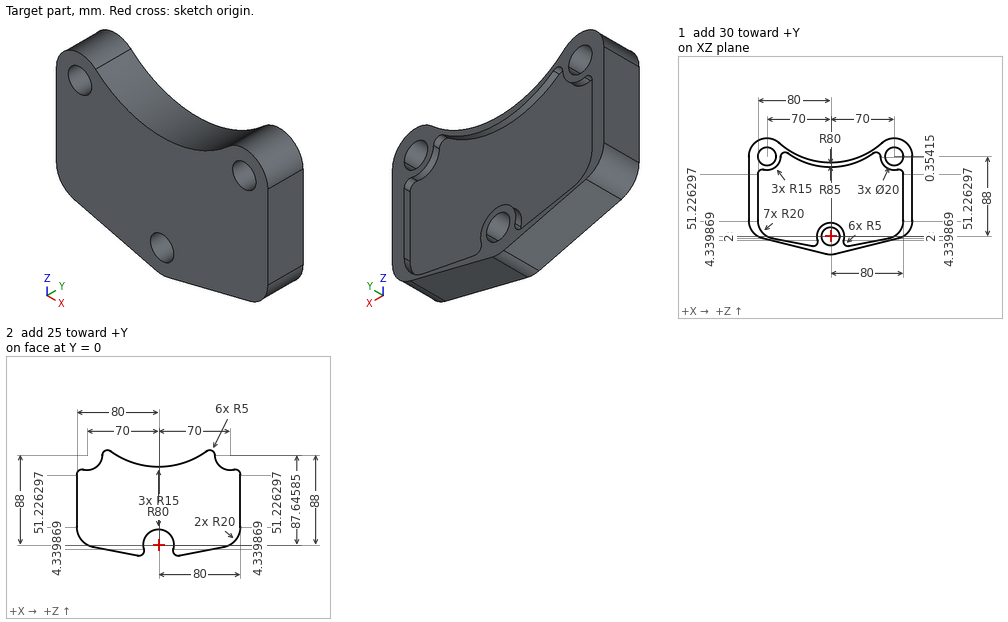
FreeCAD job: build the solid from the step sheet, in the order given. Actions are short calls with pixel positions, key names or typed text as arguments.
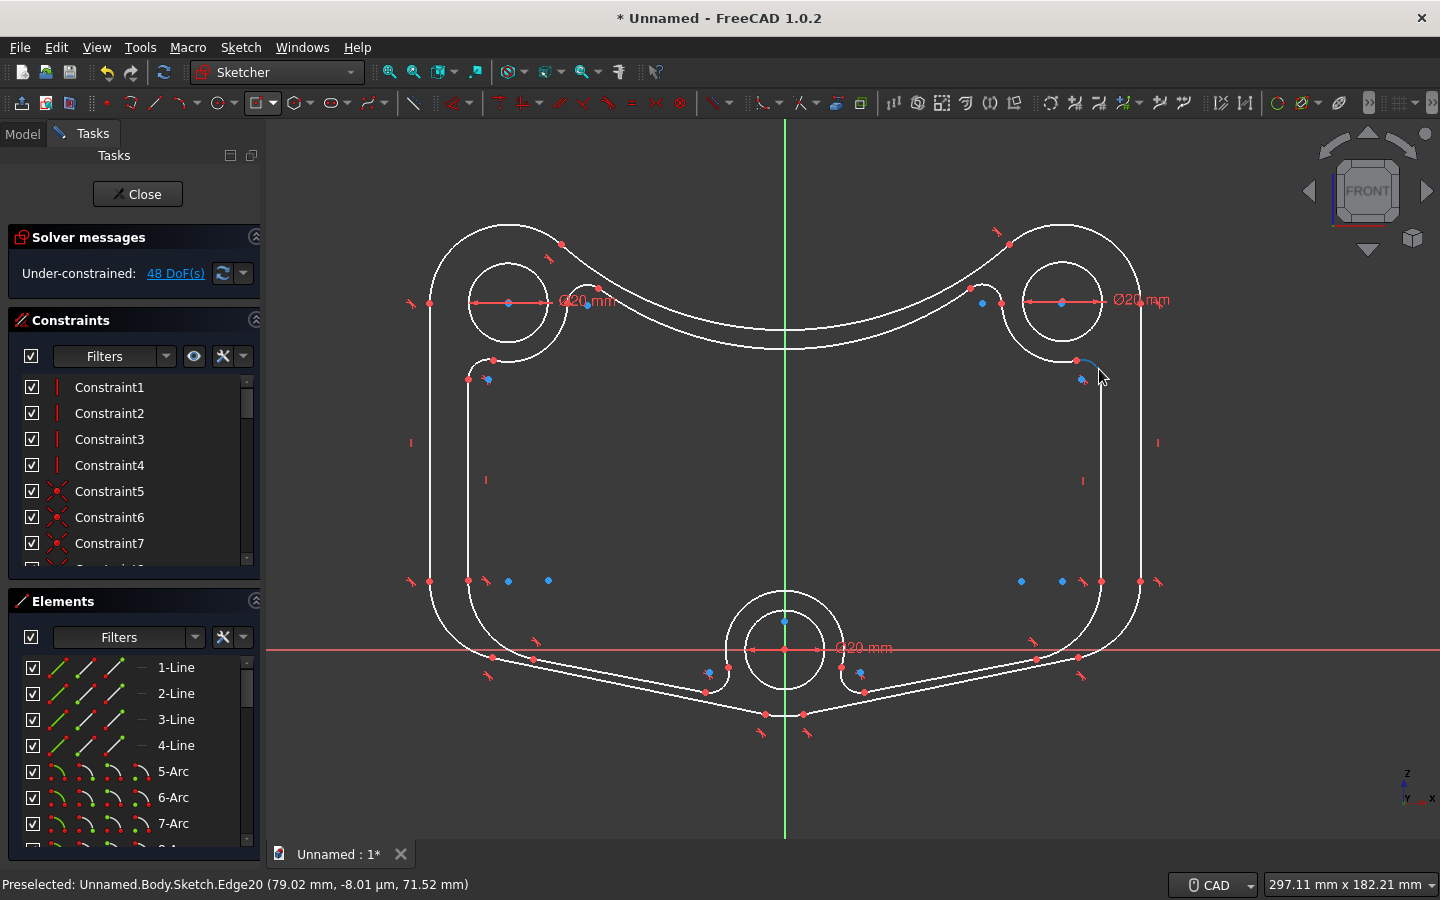
click(717, 691)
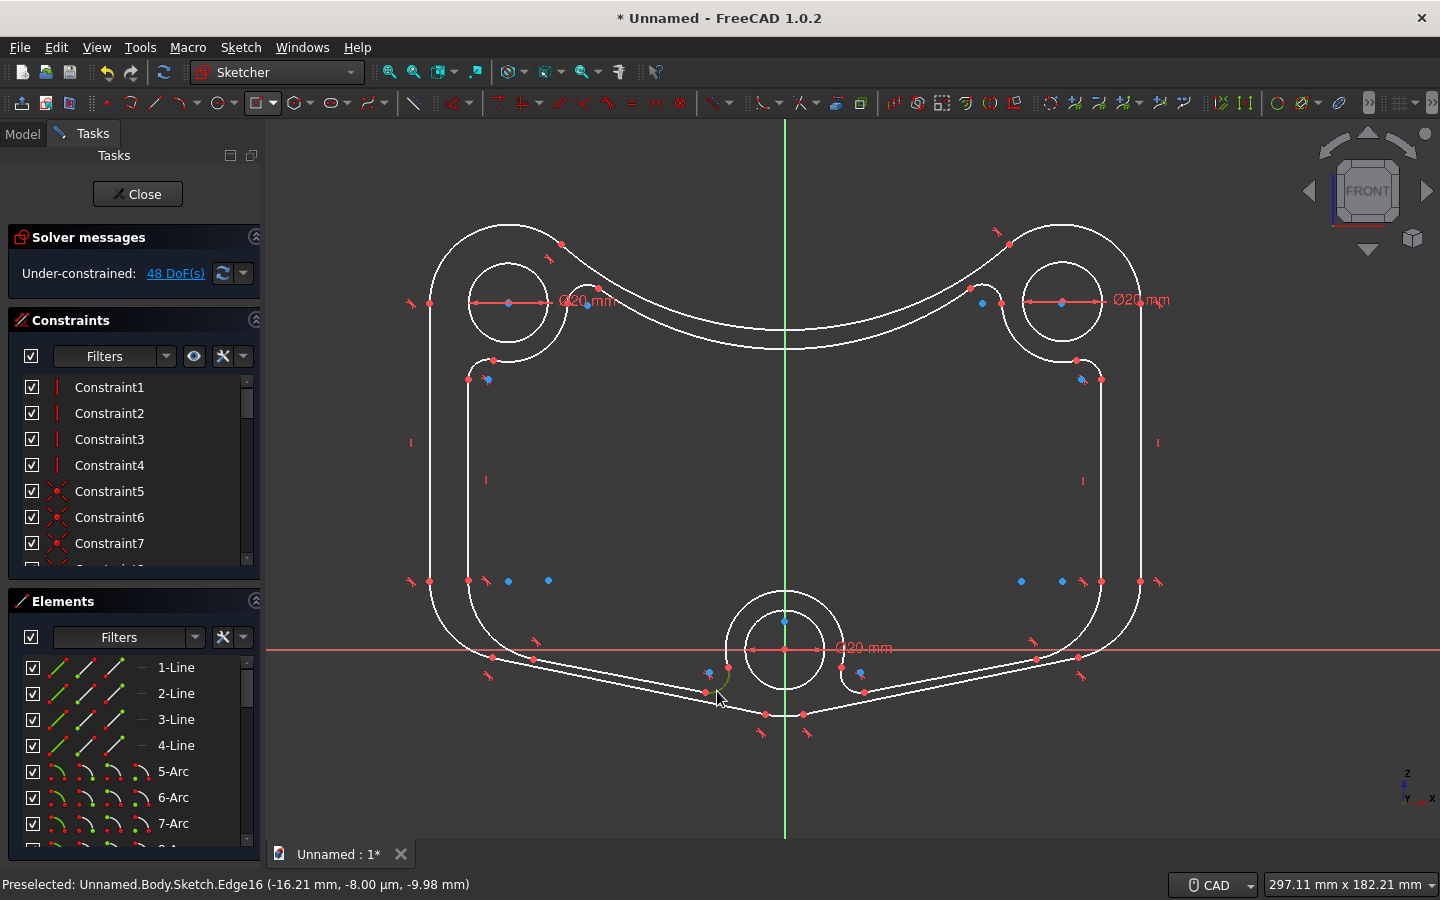
click(825, 607)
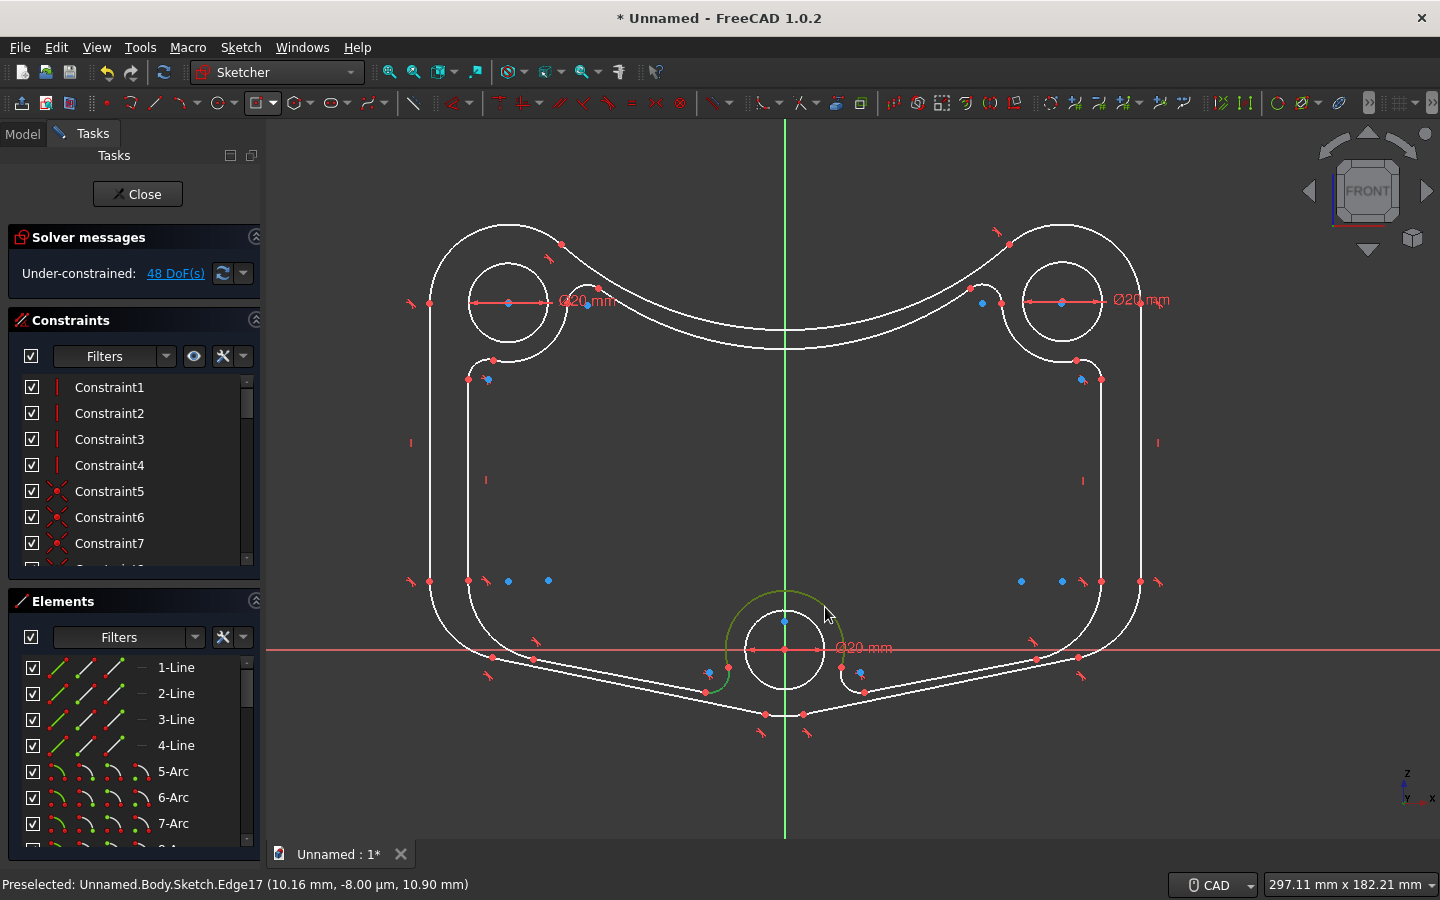
key(t)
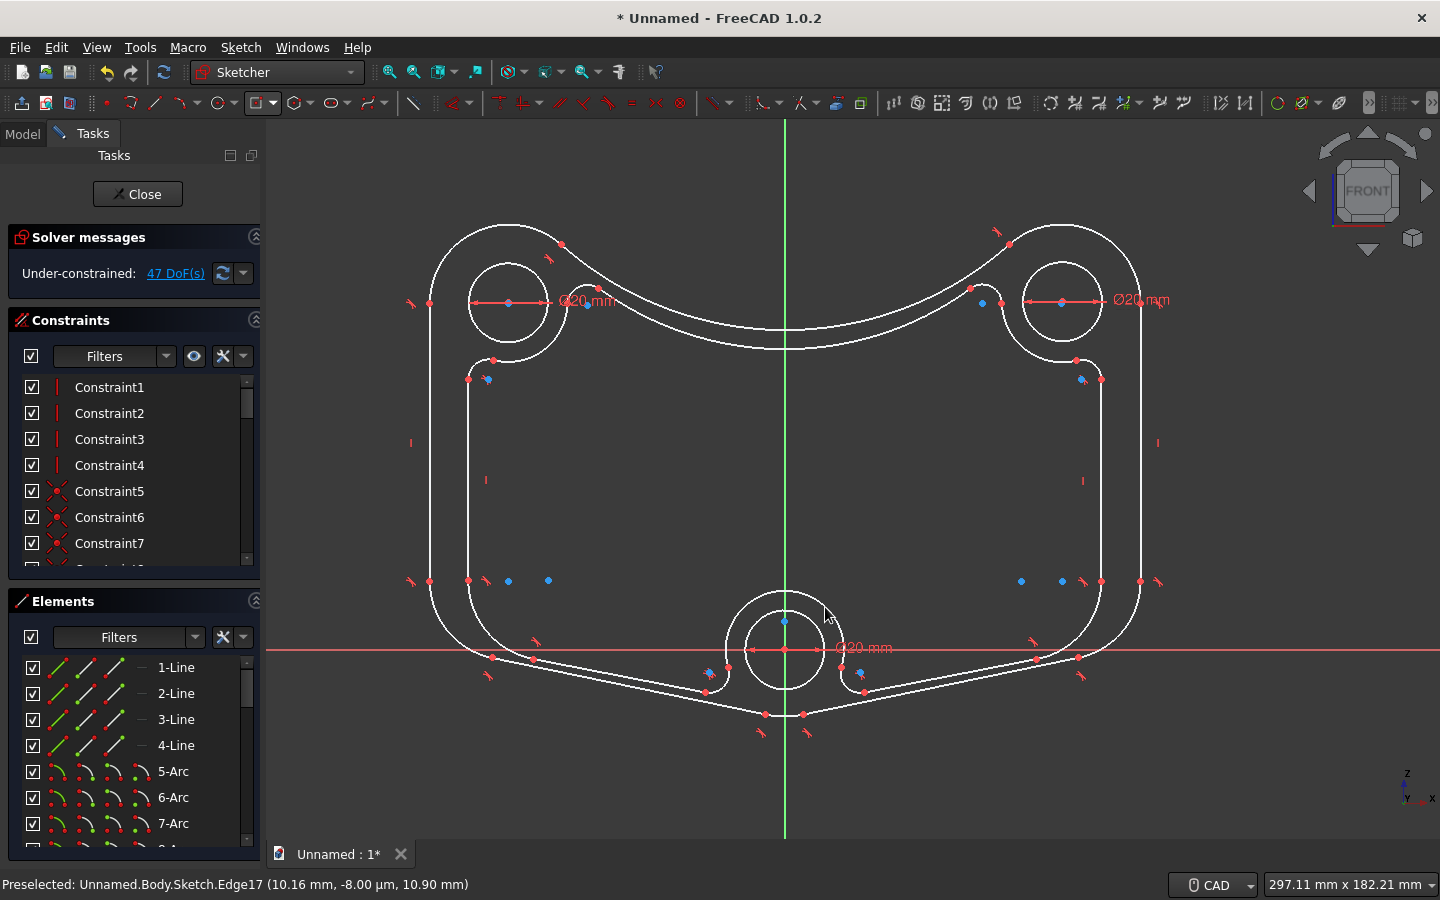
click(825, 607)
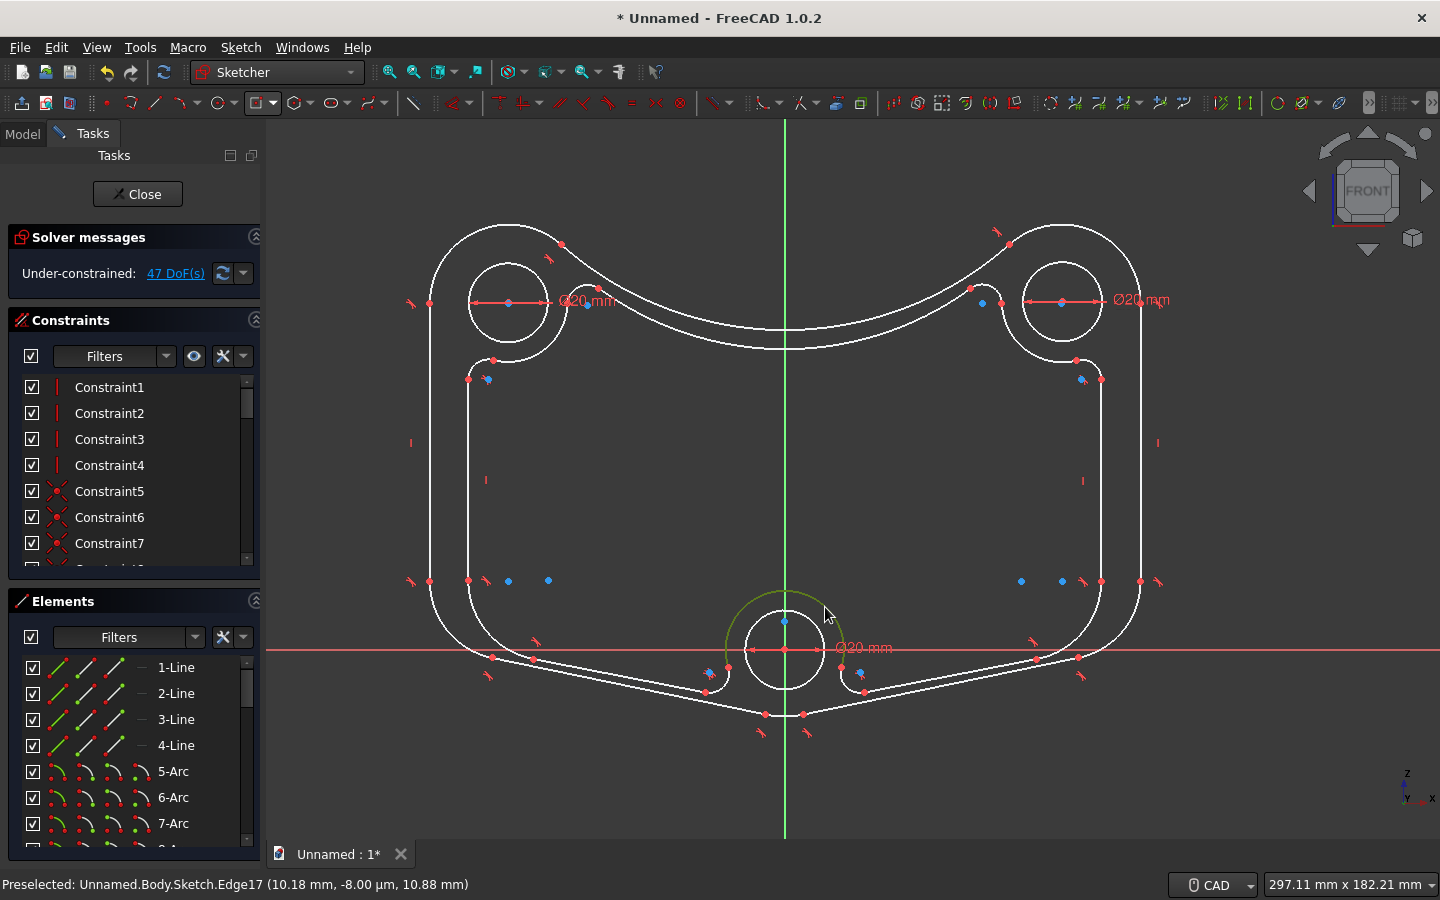
click(842, 679)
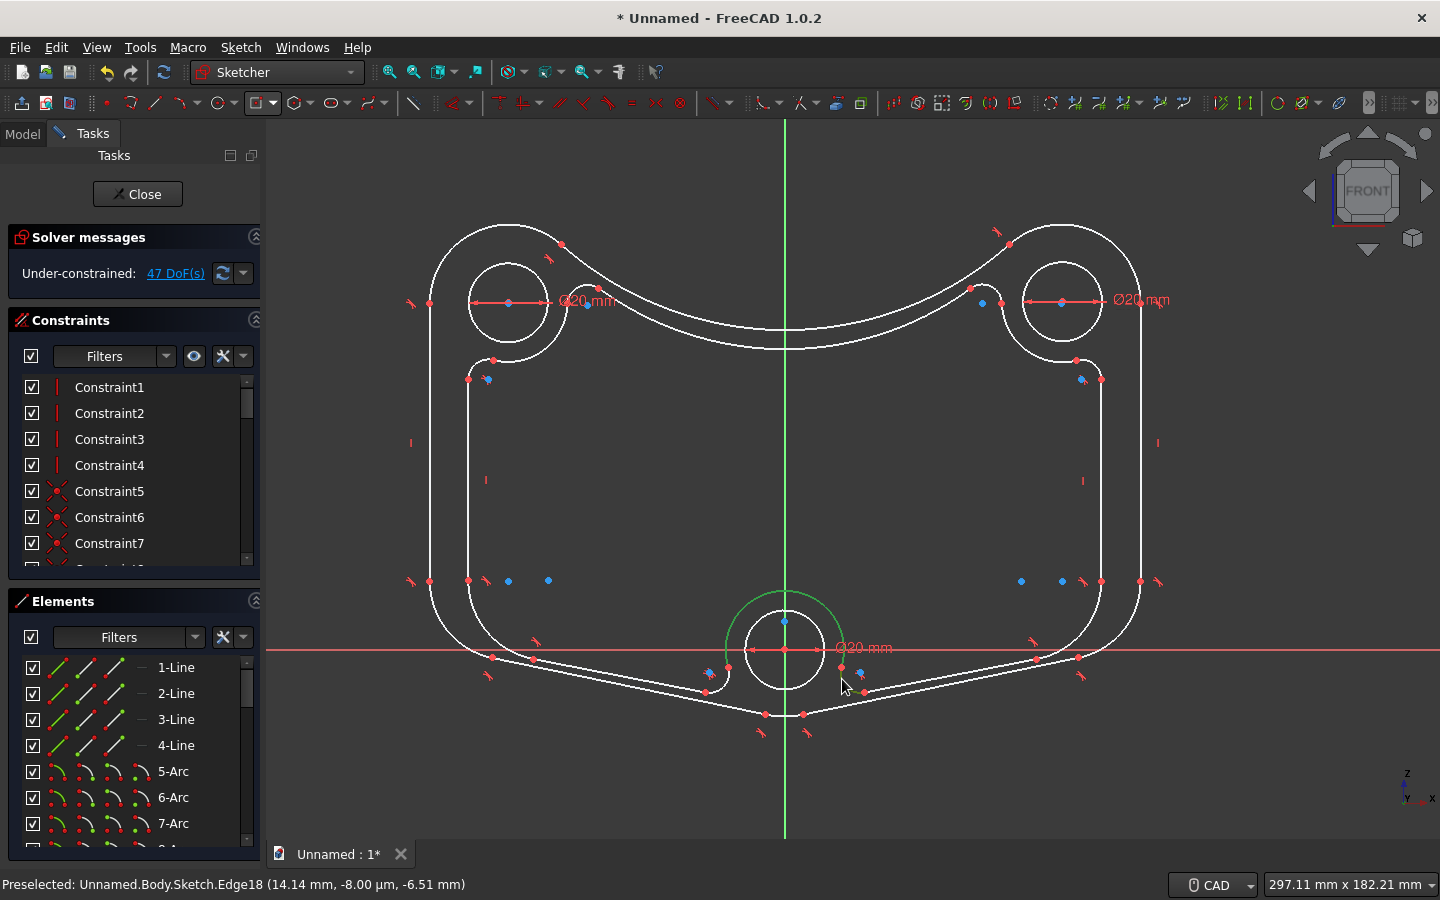
click(608, 104)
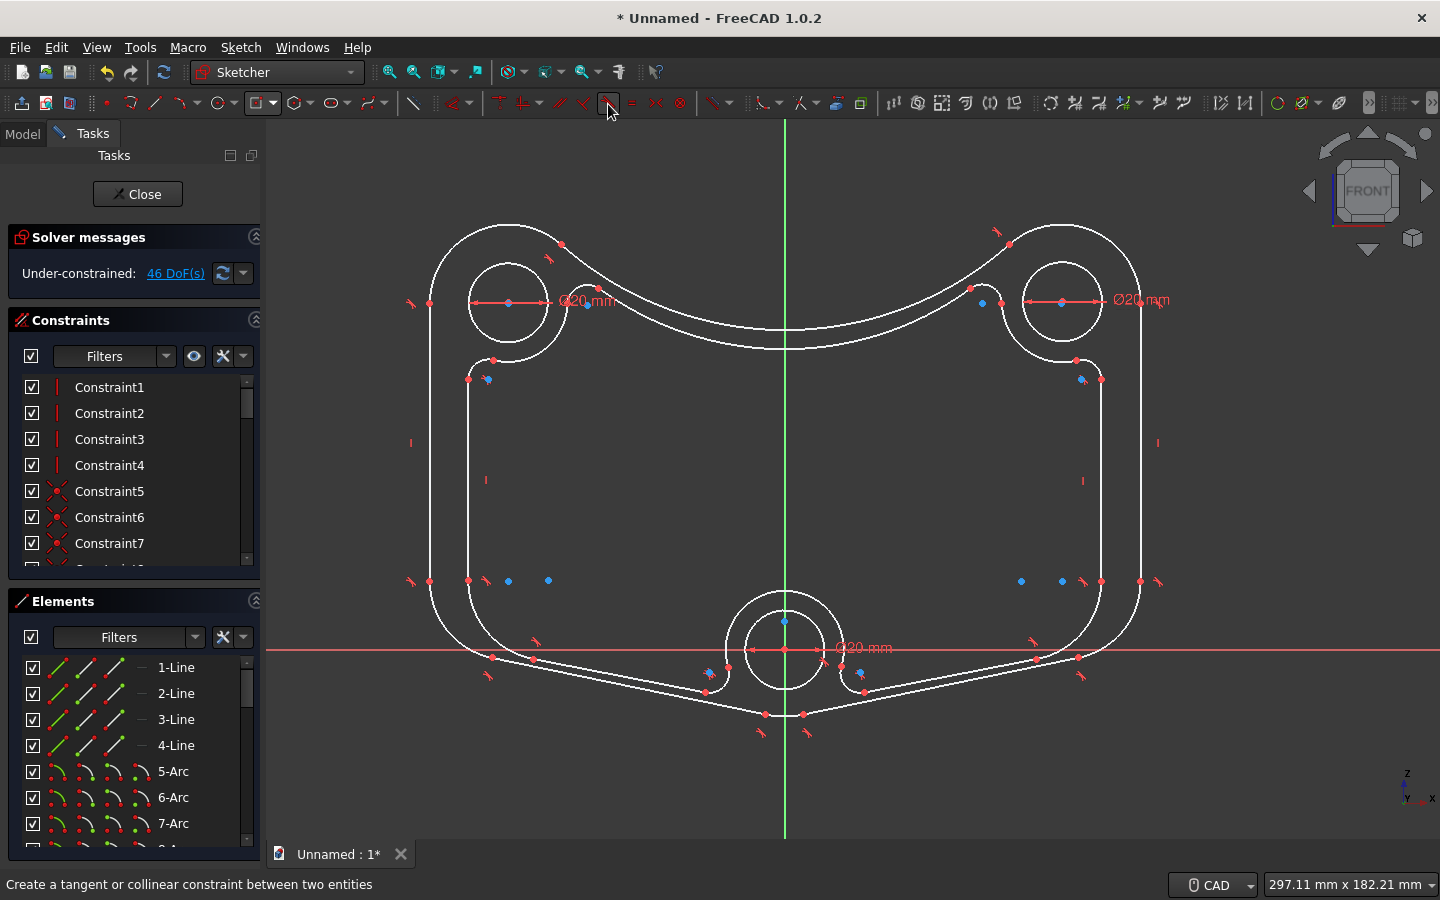
scroll(1098, 369, up, 2)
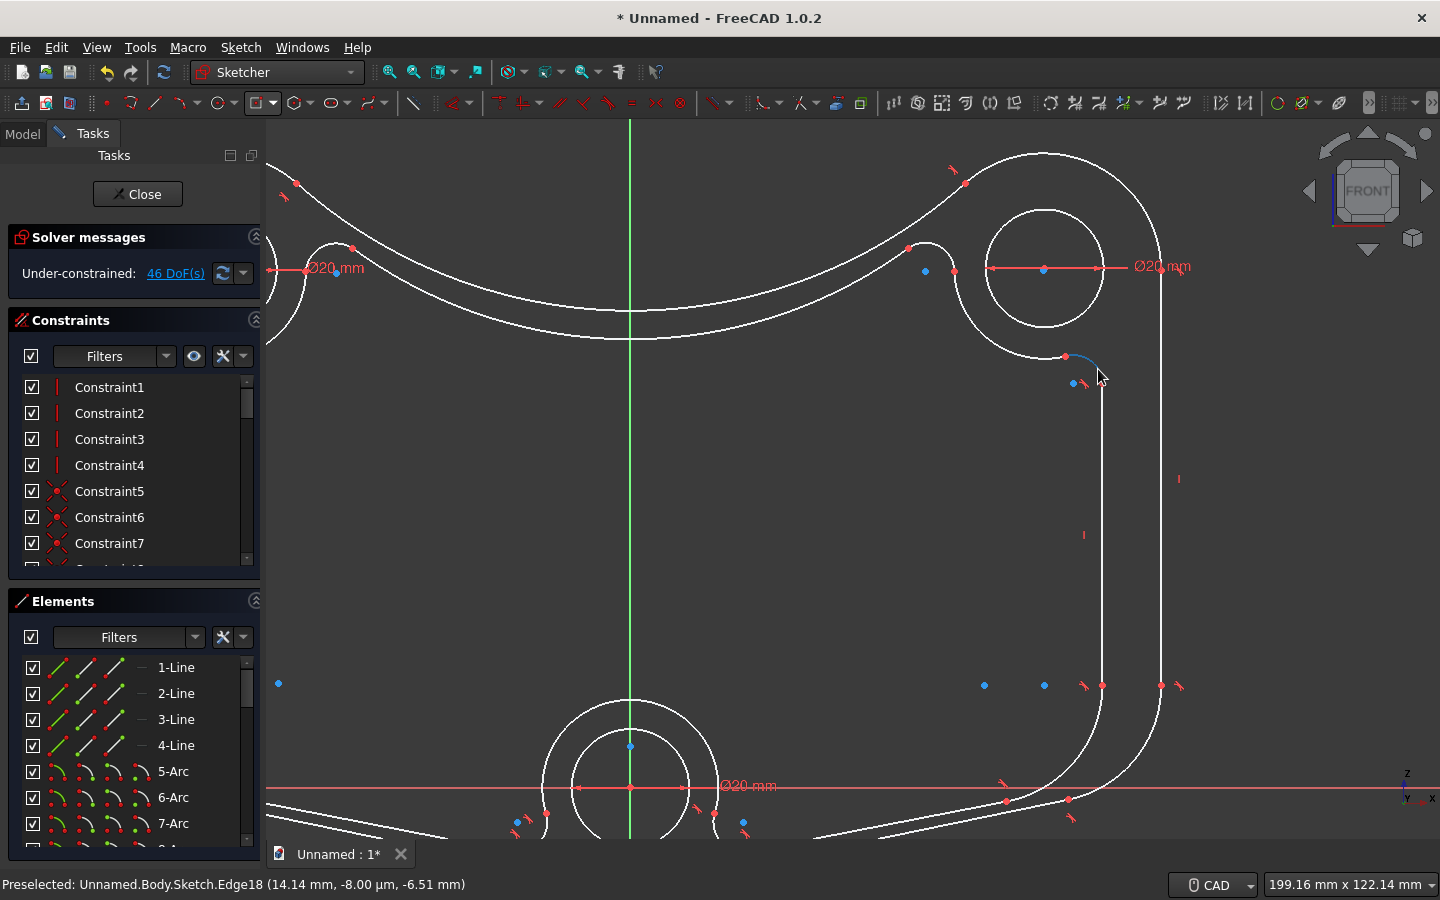
click(1098, 369)